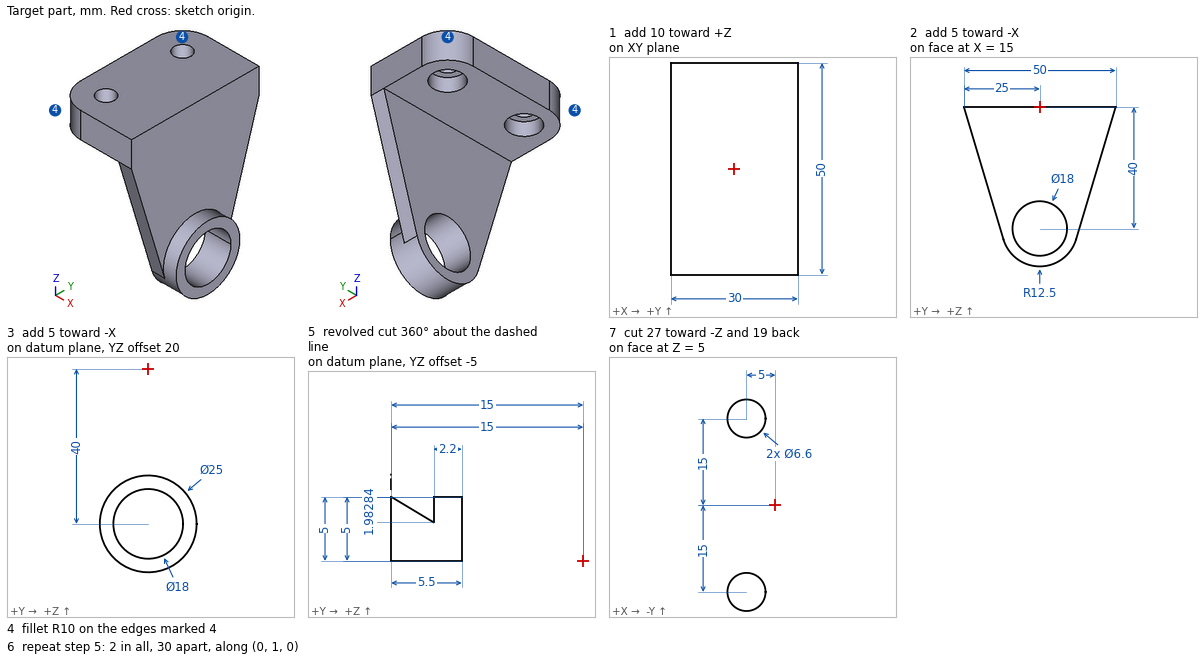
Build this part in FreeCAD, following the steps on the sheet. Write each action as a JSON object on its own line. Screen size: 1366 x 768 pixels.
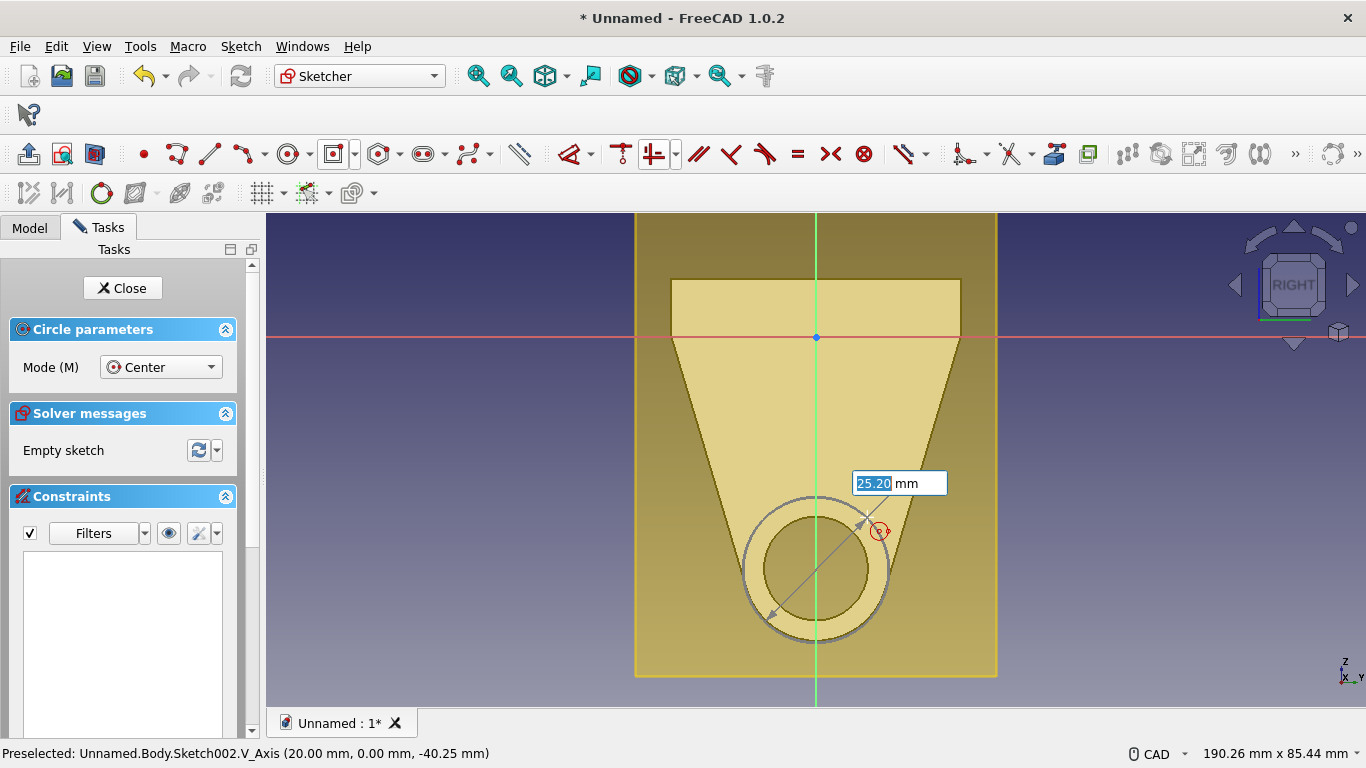
{"action": "type", "text": "25"}
{"action": "key", "text": "Return"}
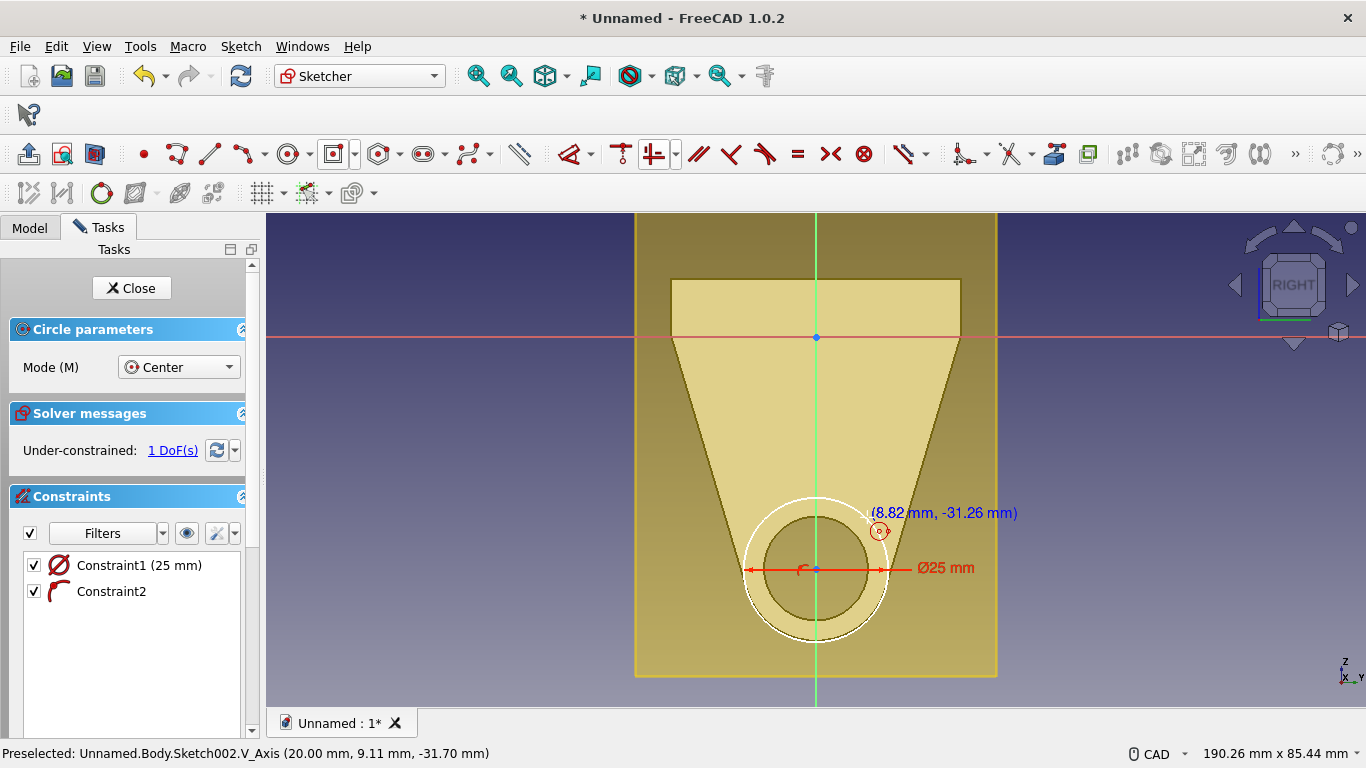
{"action": "left_click", "coordinate": [816, 570]}
{"action": "mouse_move", "coordinate": [853, 532]}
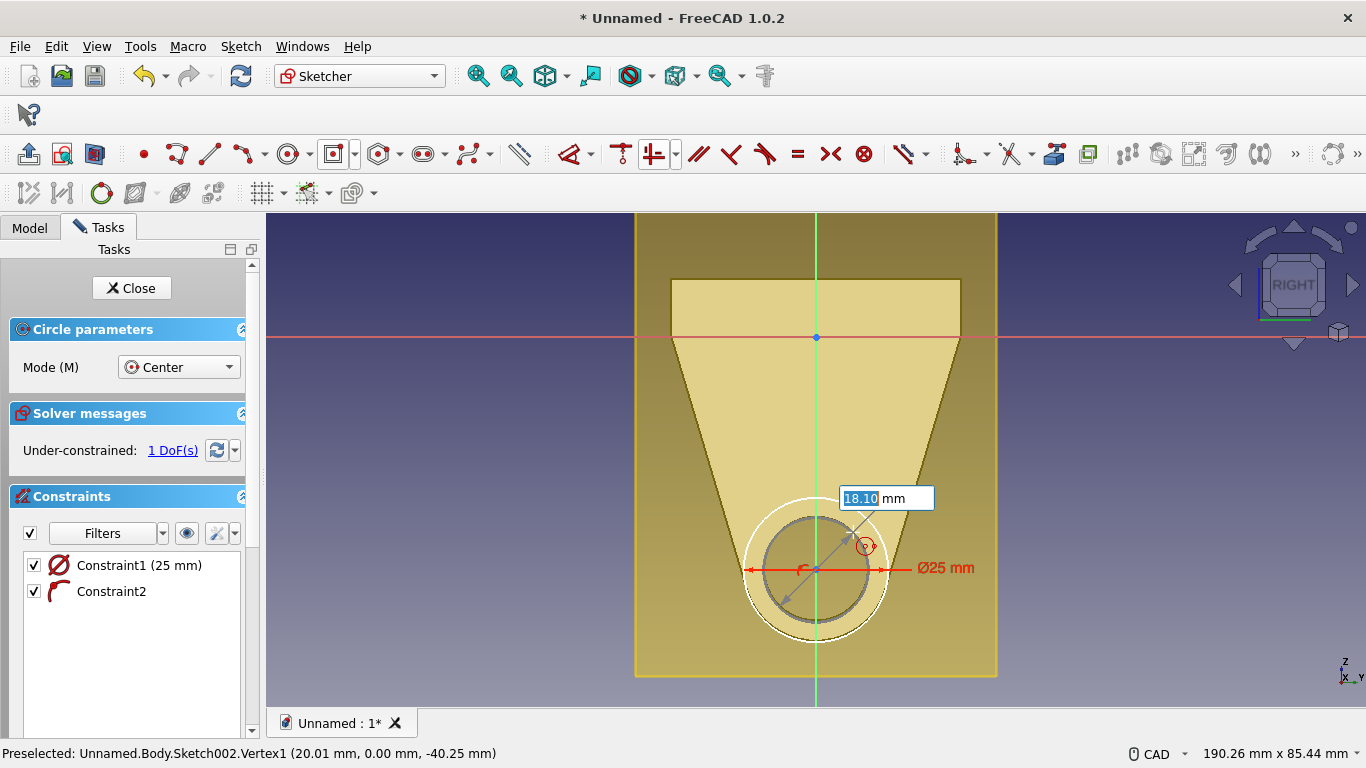
{"action": "type", "text": "18"}
{"action": "key", "text": "Return"}
{"action": "key", "text": "Escape"}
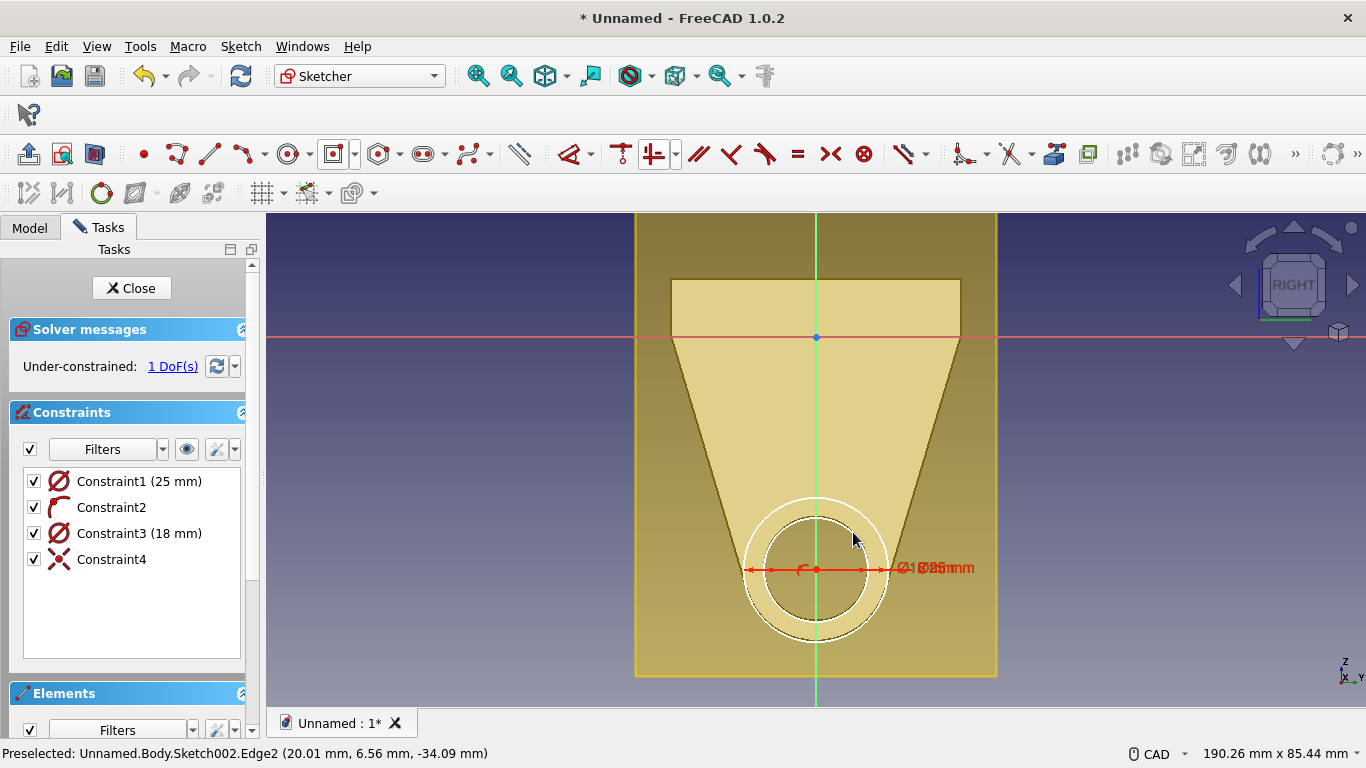
{"action": "left_click", "coordinate": [568, 154]}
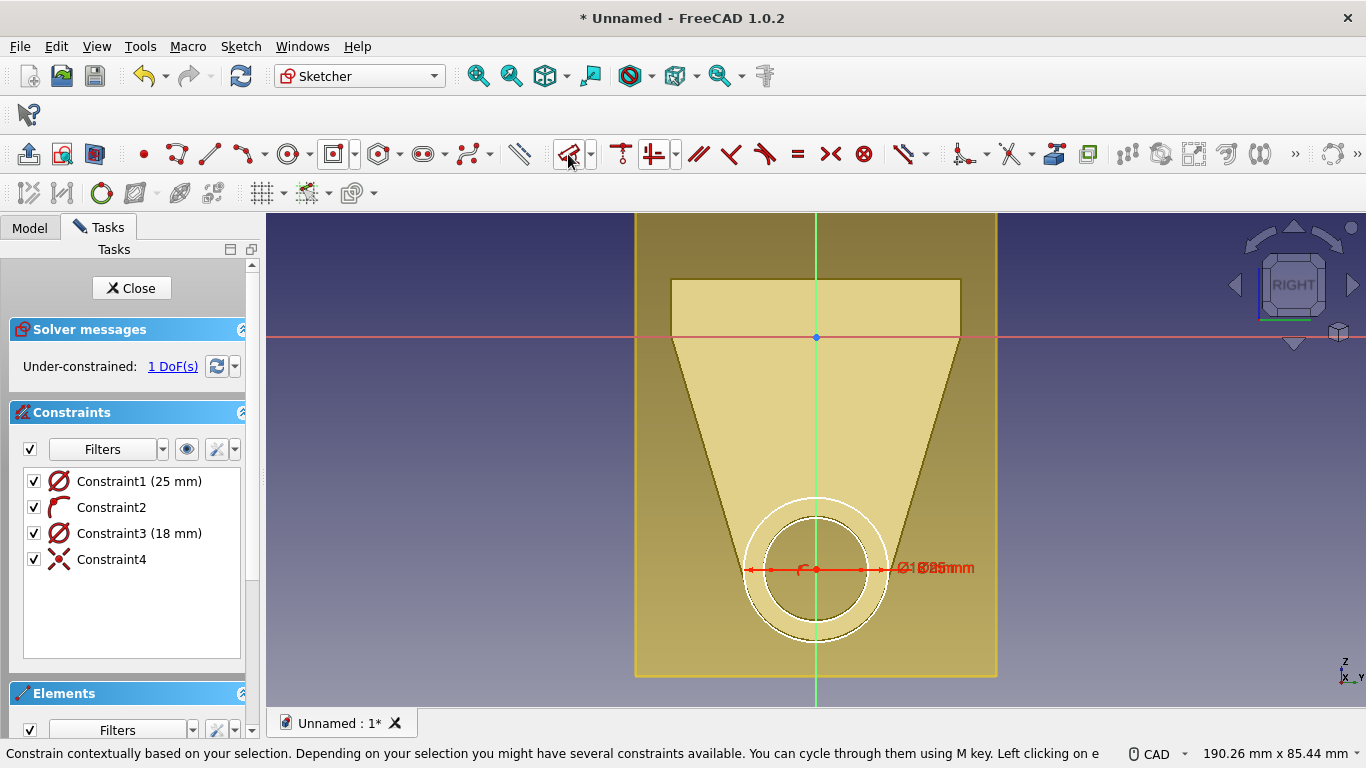
{"action": "left_click", "coordinate": [816, 570]}
{"action": "left_click", "coordinate": [850, 454]}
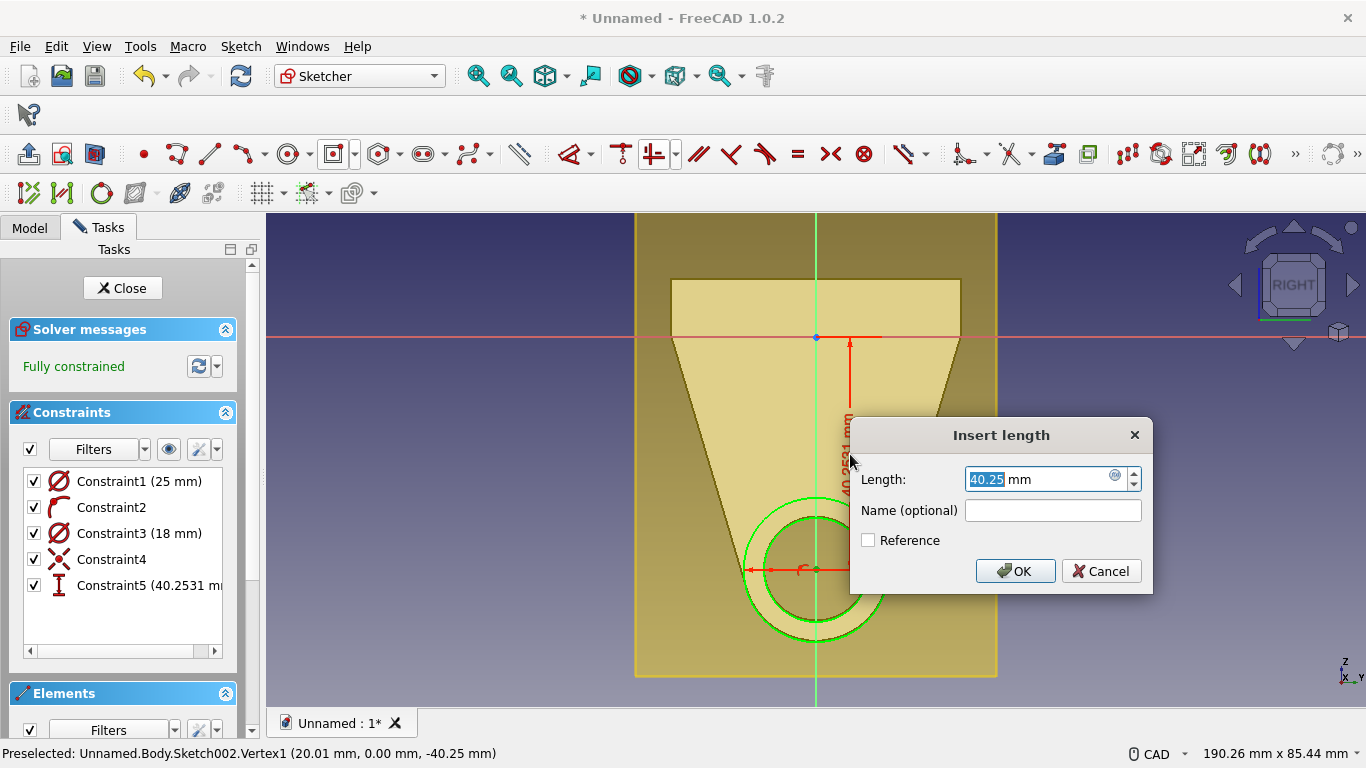
{"action": "type", "text": "40"}
{"action": "key", "text": "Return"}
{"action": "key", "text": "Escape"}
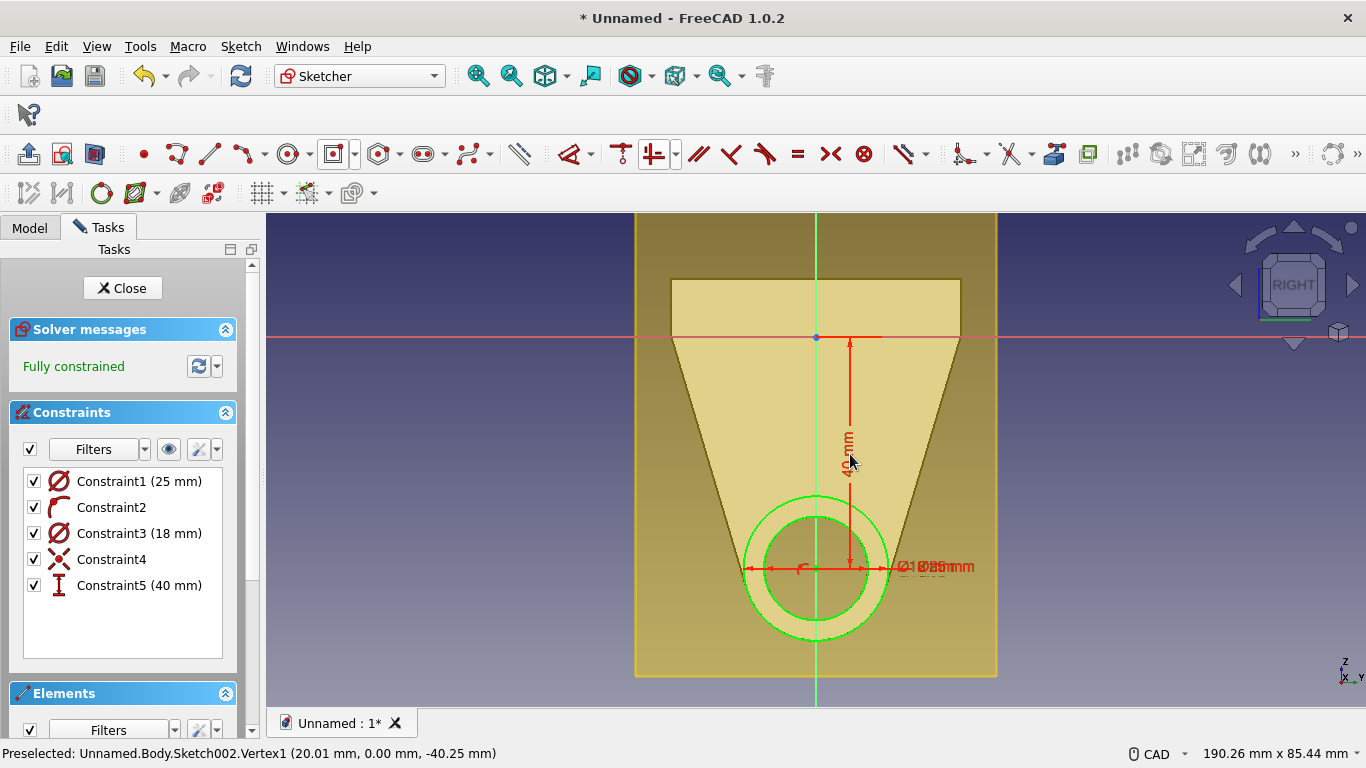
{"action": "left_click", "coordinate": [123, 288]}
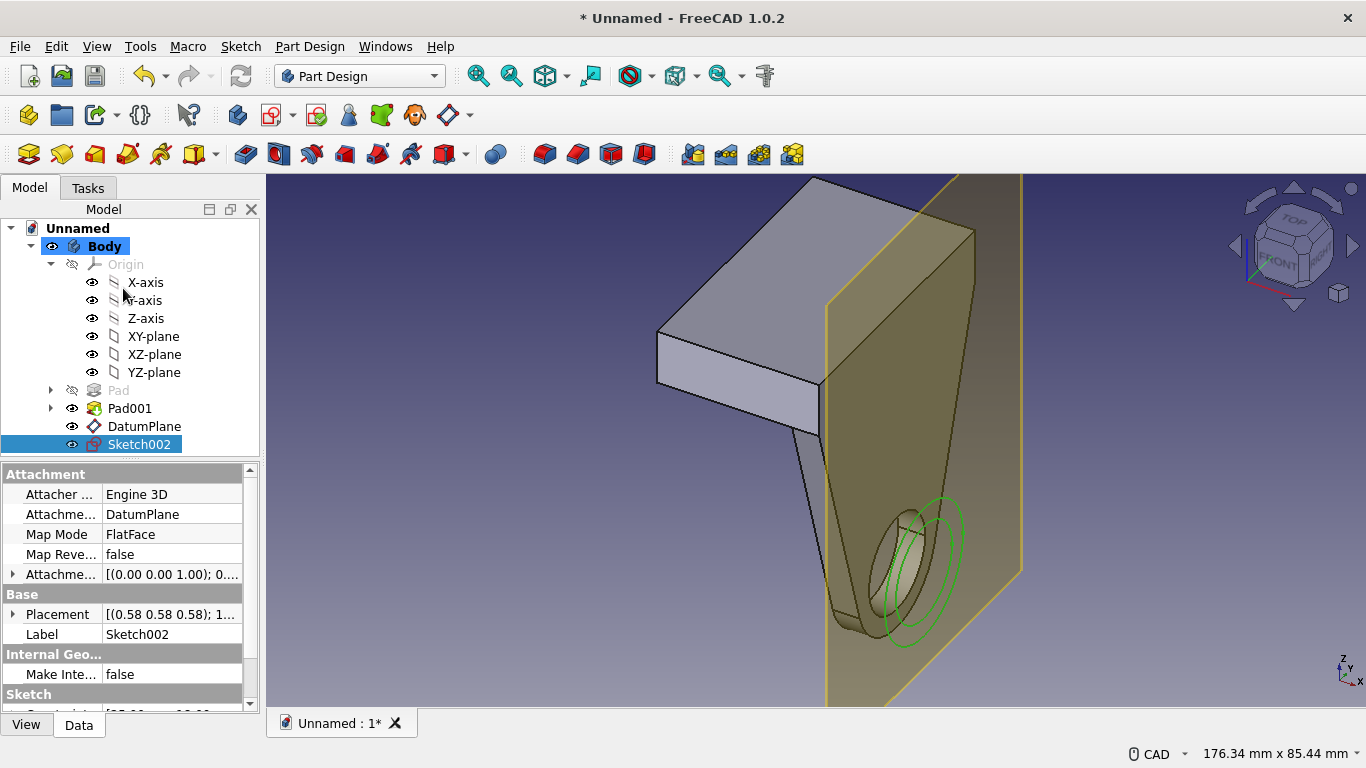
{"action": "left_click", "coordinate": [29, 154]}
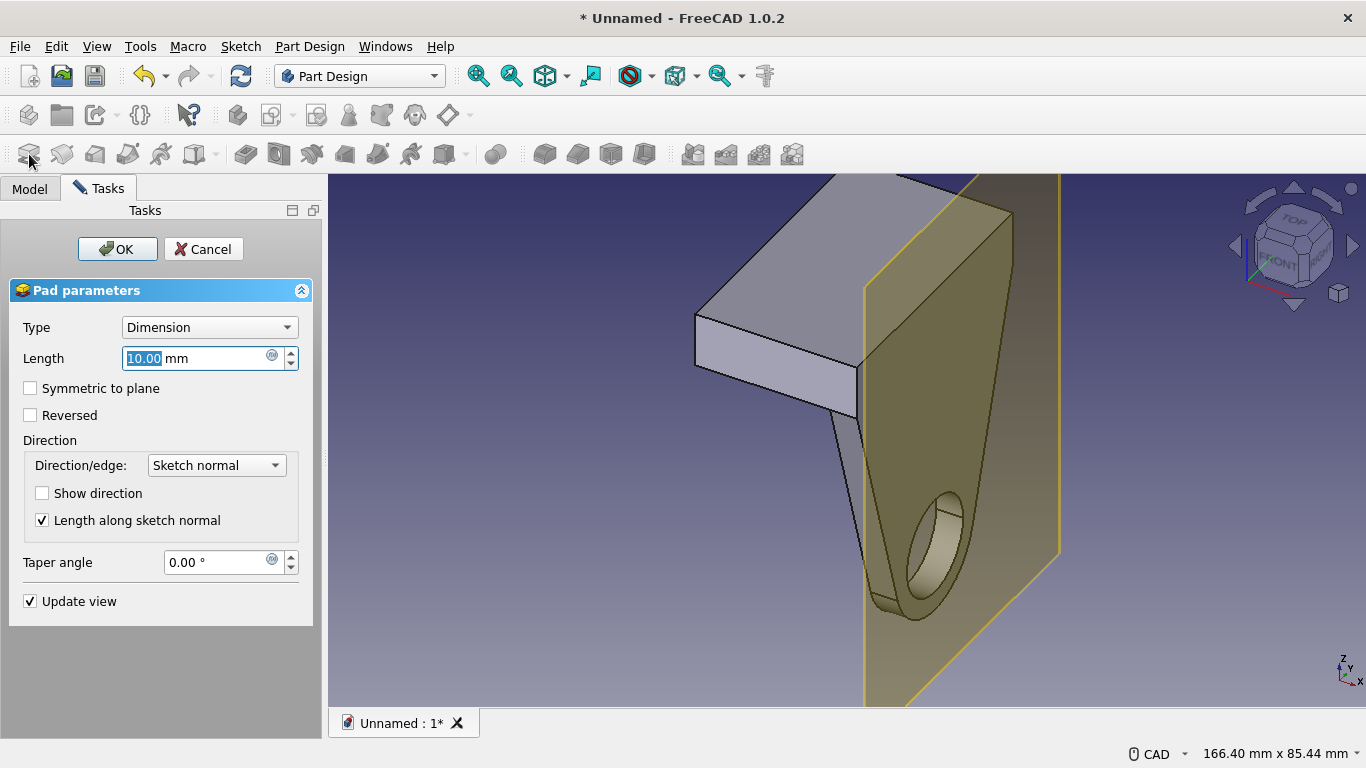
{"action": "type", "text": "5"}
{"action": "key", "text": "Tab"}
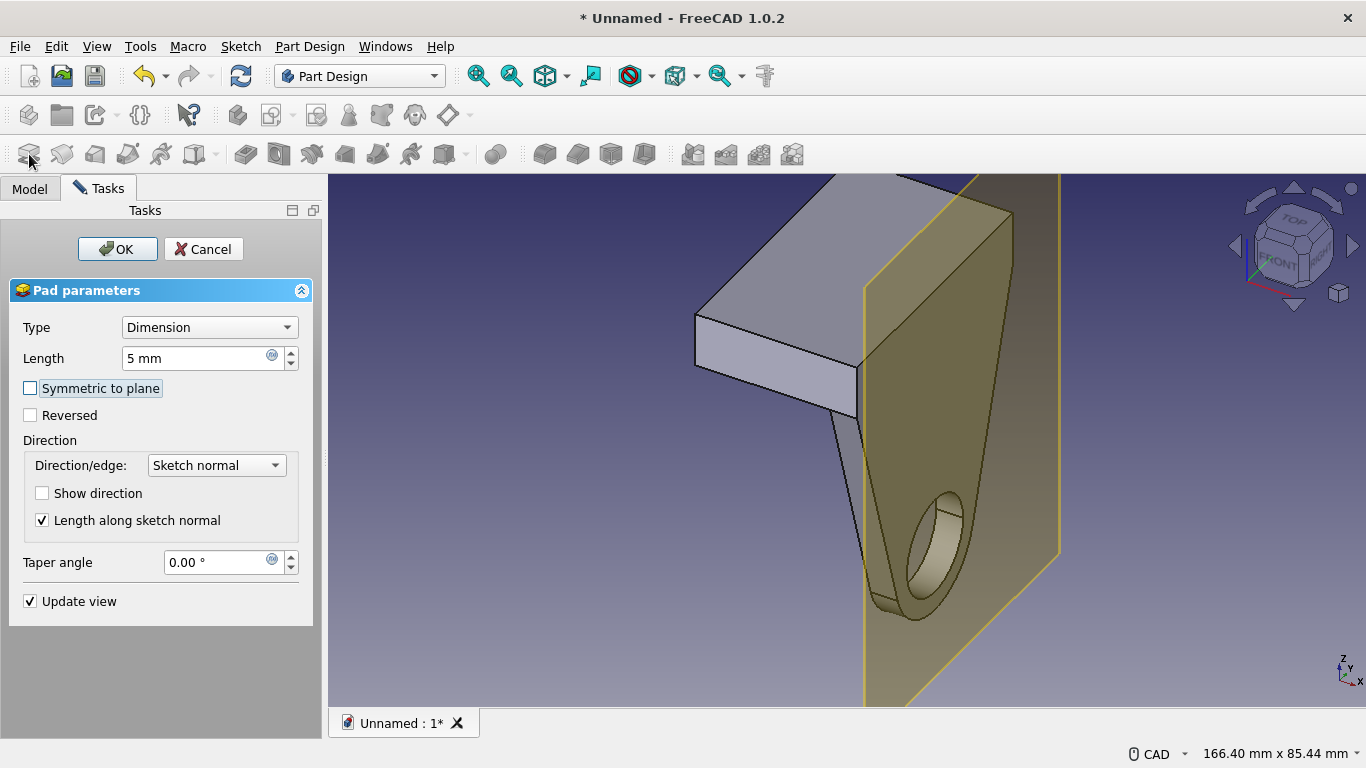
{"action": "left_click", "coordinate": [31, 415]}